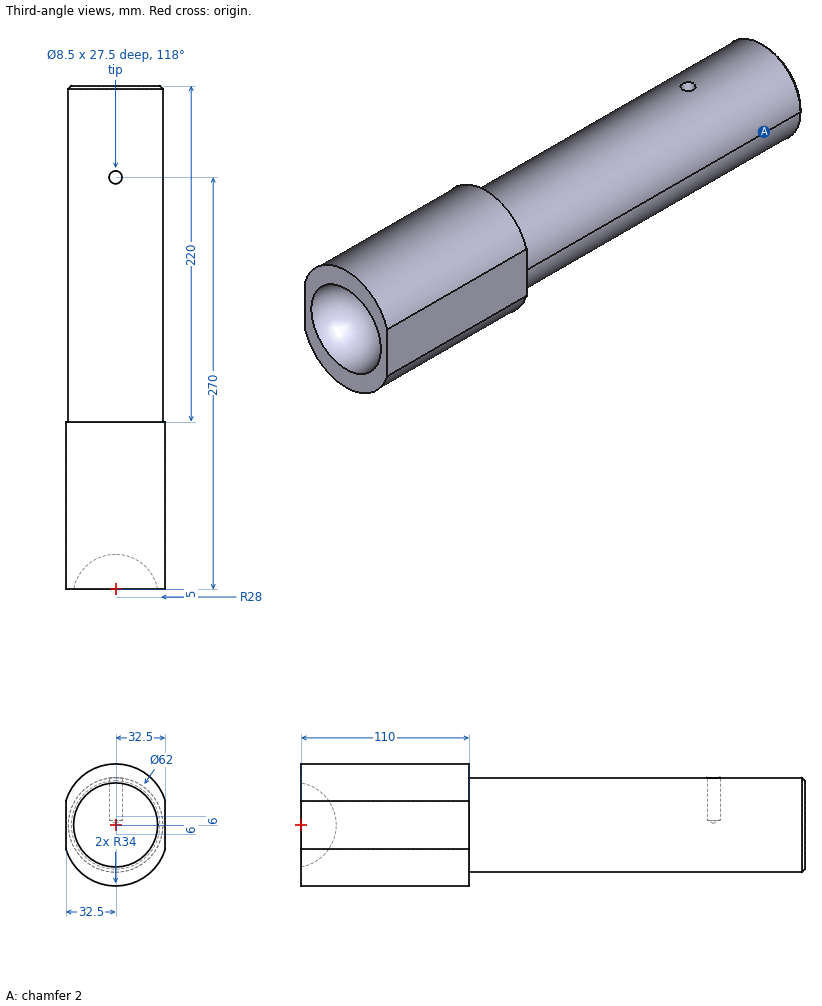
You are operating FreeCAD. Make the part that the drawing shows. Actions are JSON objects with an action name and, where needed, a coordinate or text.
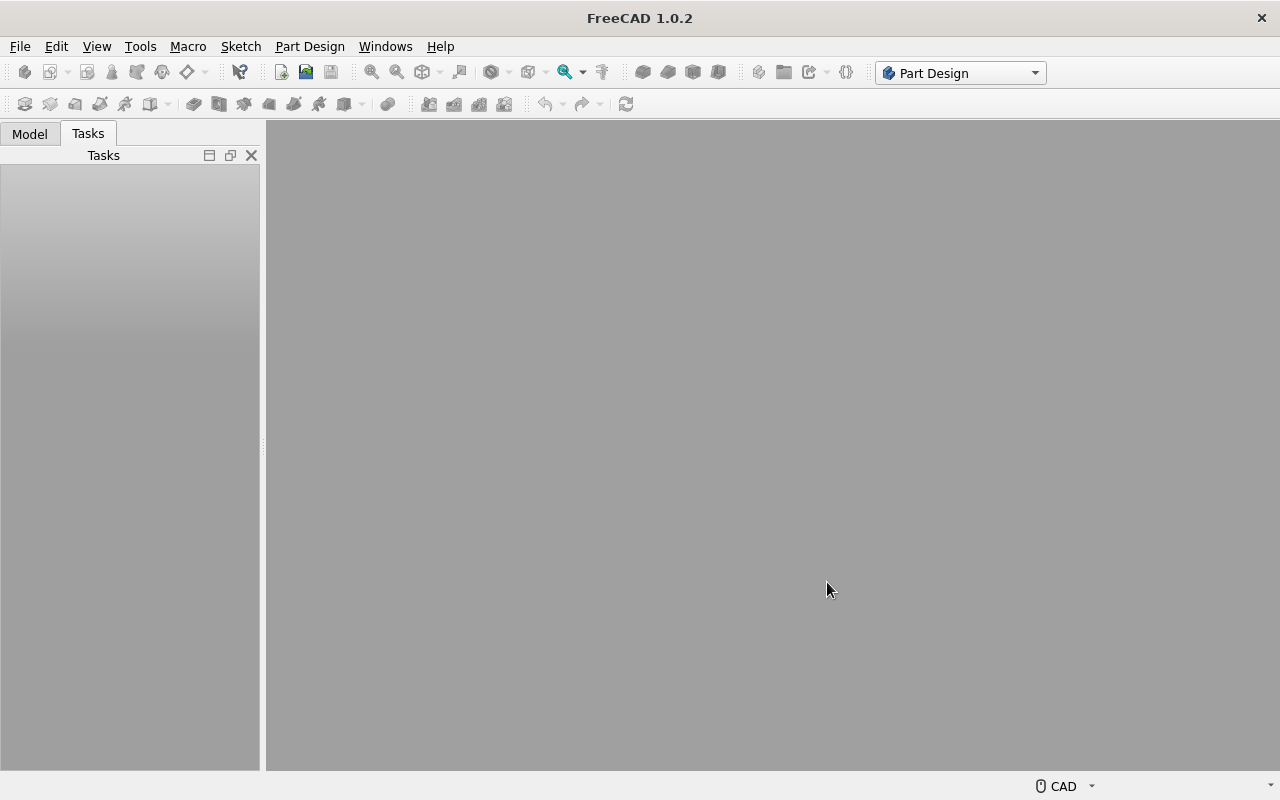
{"action": "left_click", "coordinate": [281, 72]}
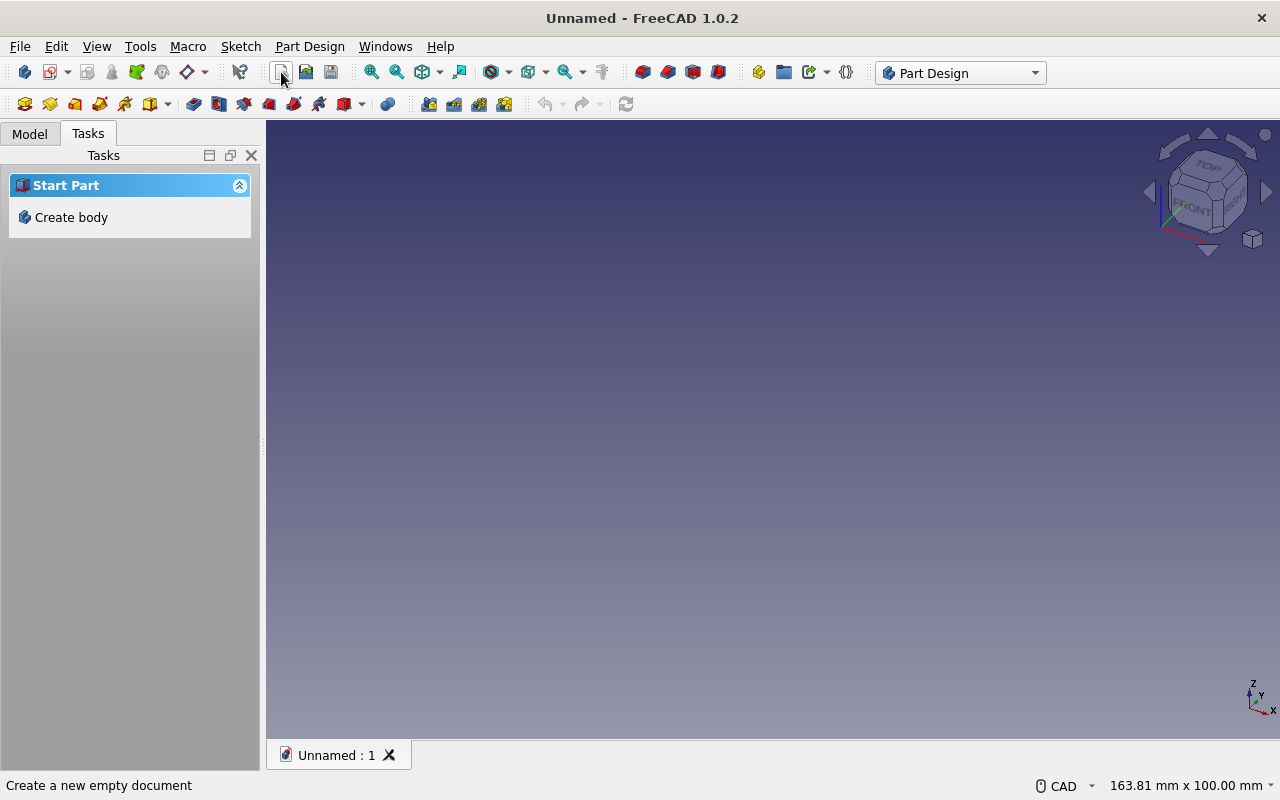
{"action": "left_click", "coordinate": [50, 72]}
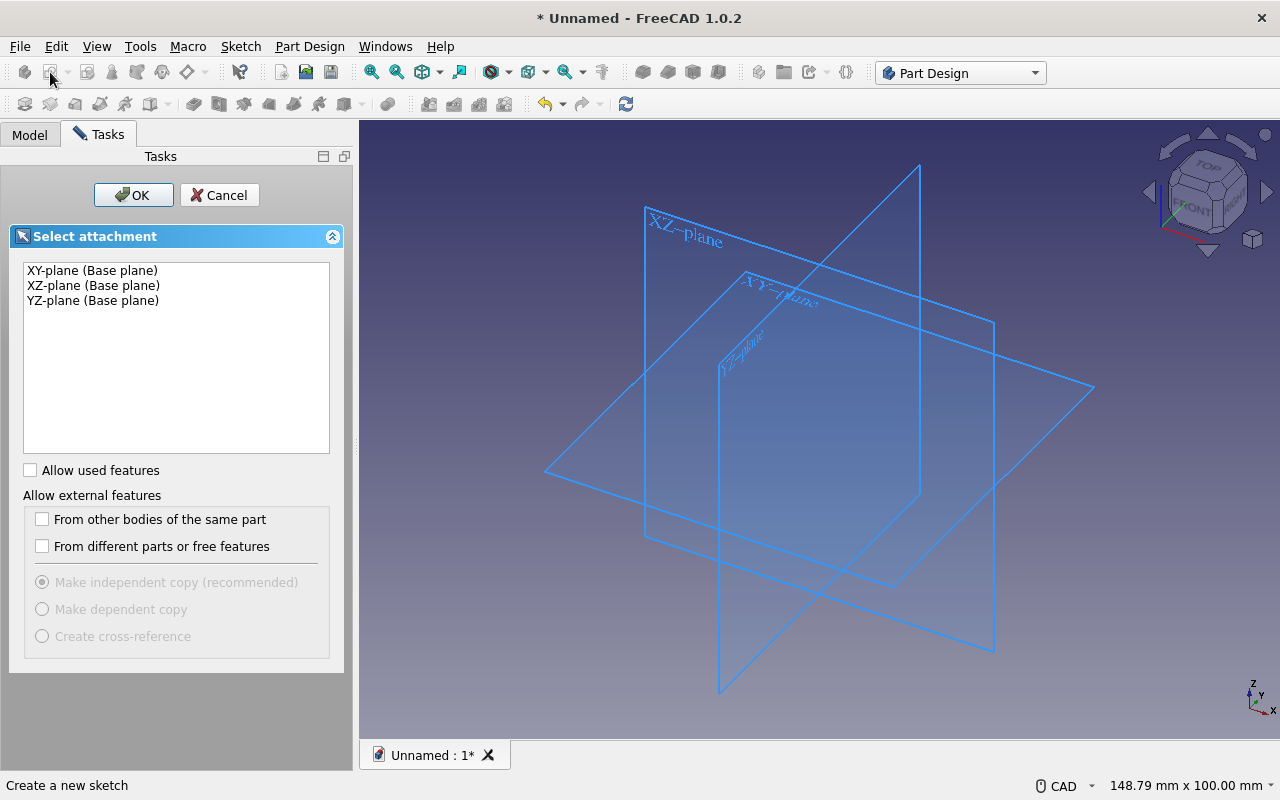
{"action": "left_click", "coordinate": [84, 286]}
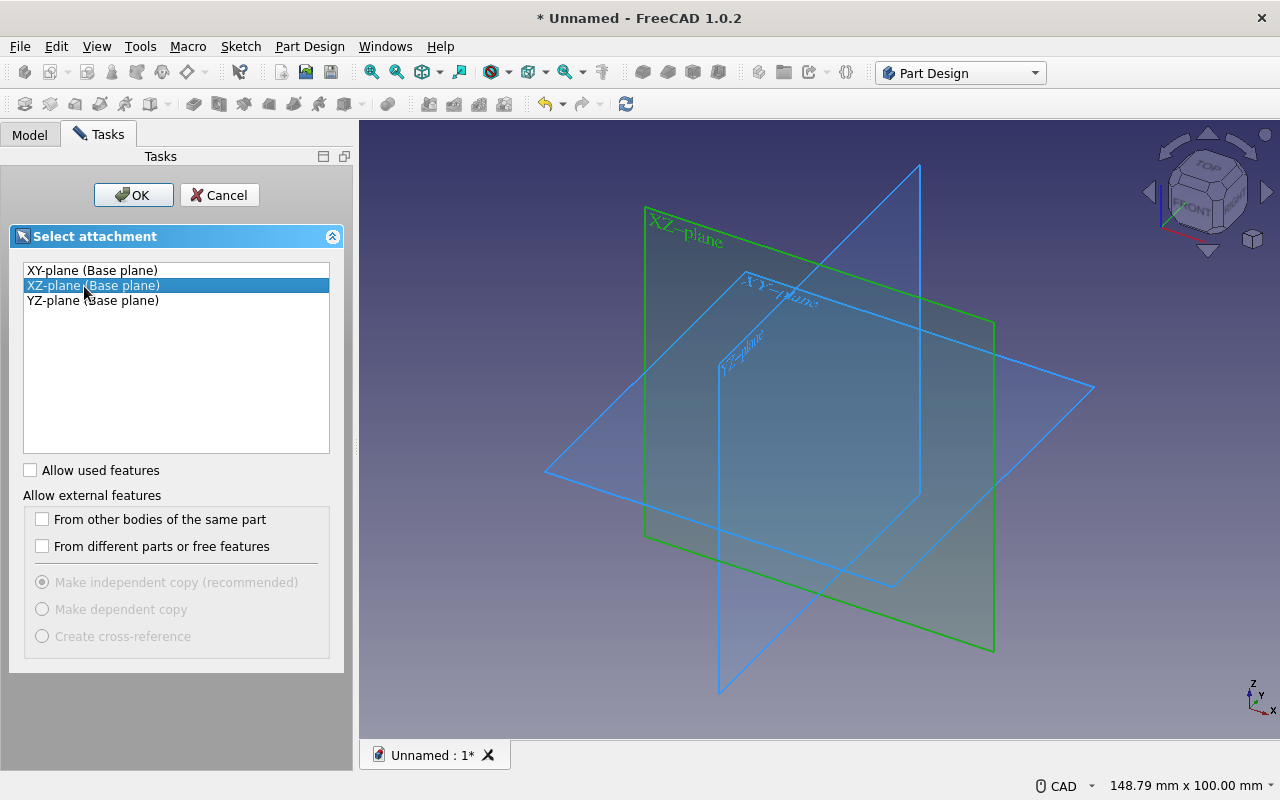
{"action": "left_click", "coordinate": [134, 195]}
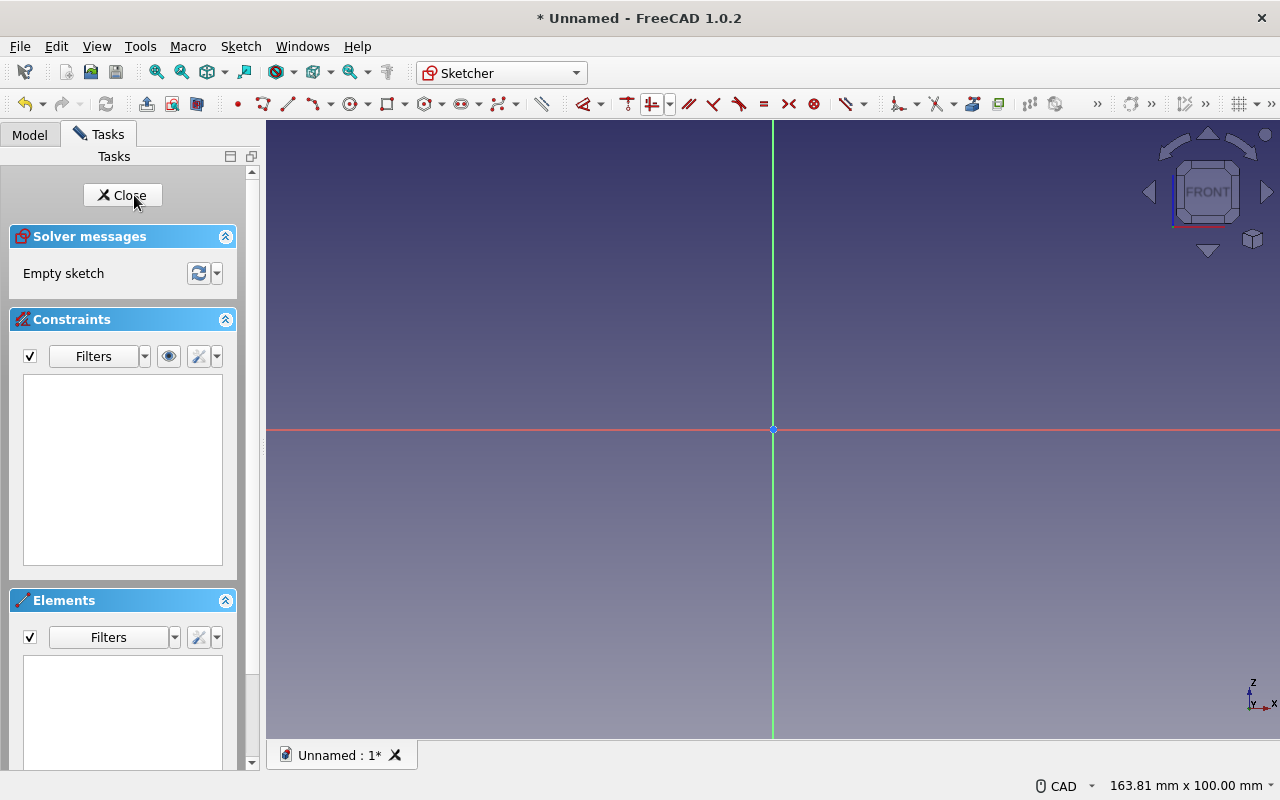
{"action": "left_click", "coordinate": [288, 104]}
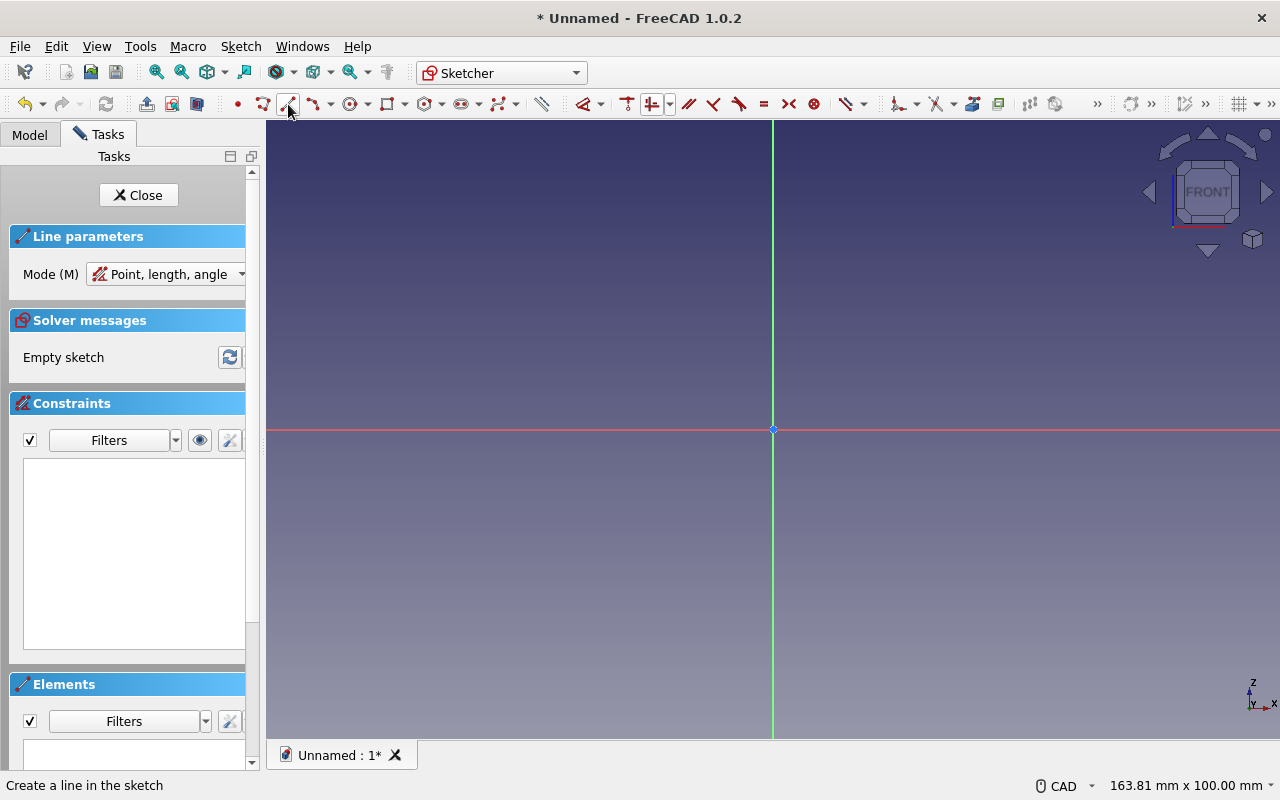
{"action": "left_click", "coordinate": [974, 331]}
{"action": "left_click", "coordinate": [974, 528]}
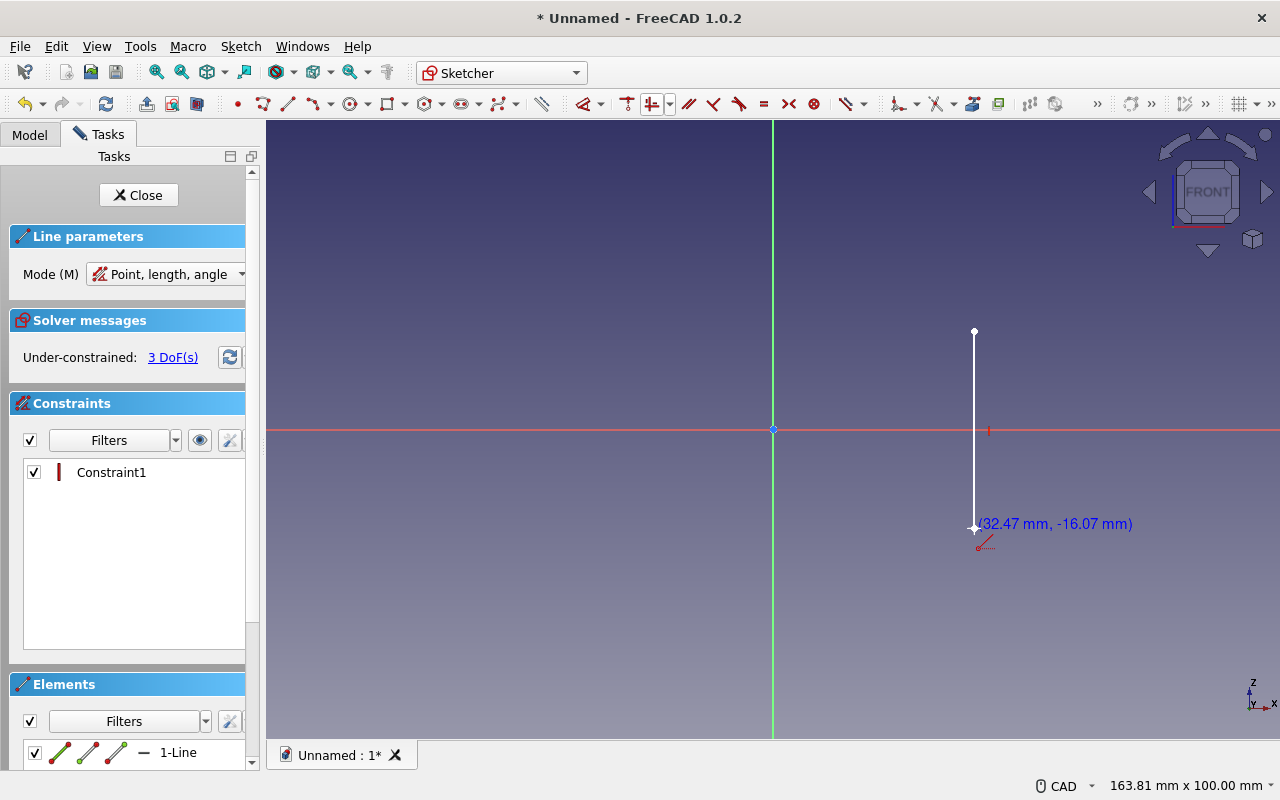
{"action": "left_click", "coordinate": [572, 528]}
{"action": "left_click", "coordinate": [572, 331]}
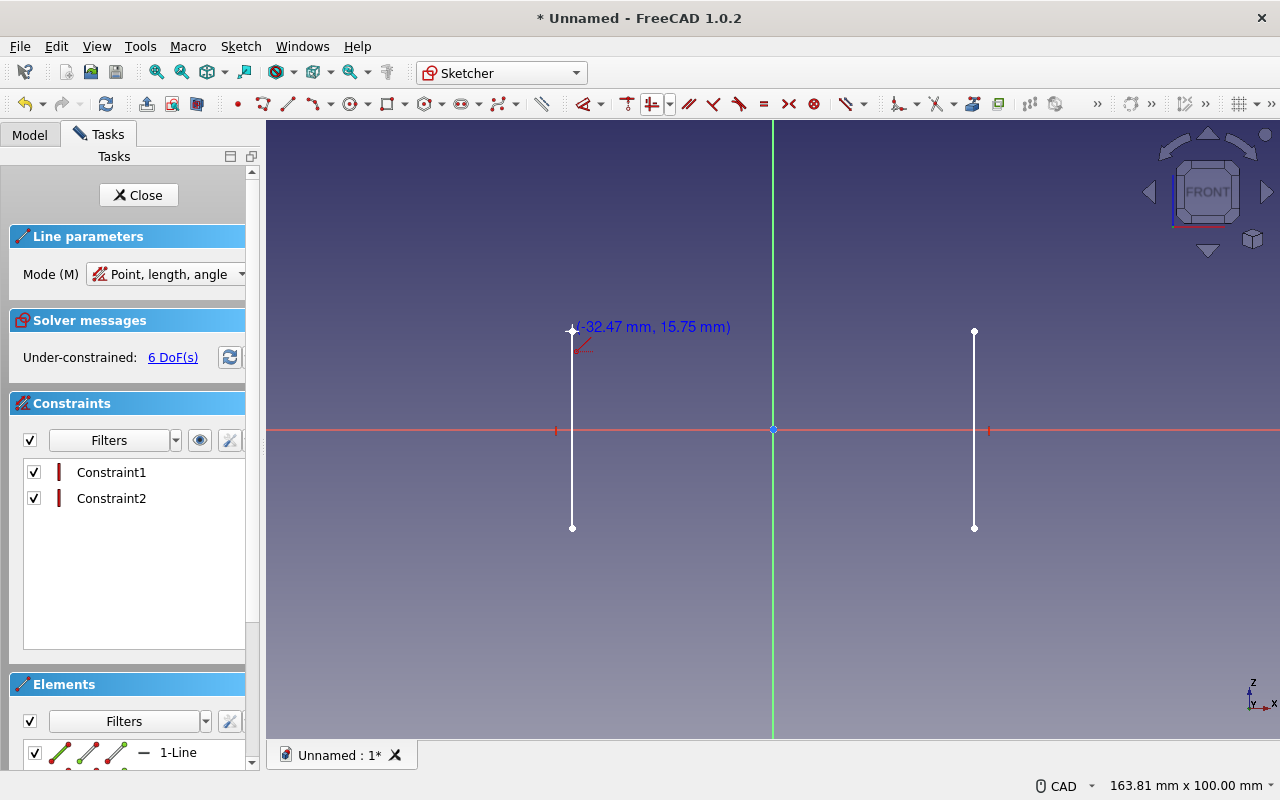
{"action": "left_click", "coordinate": [312, 104]}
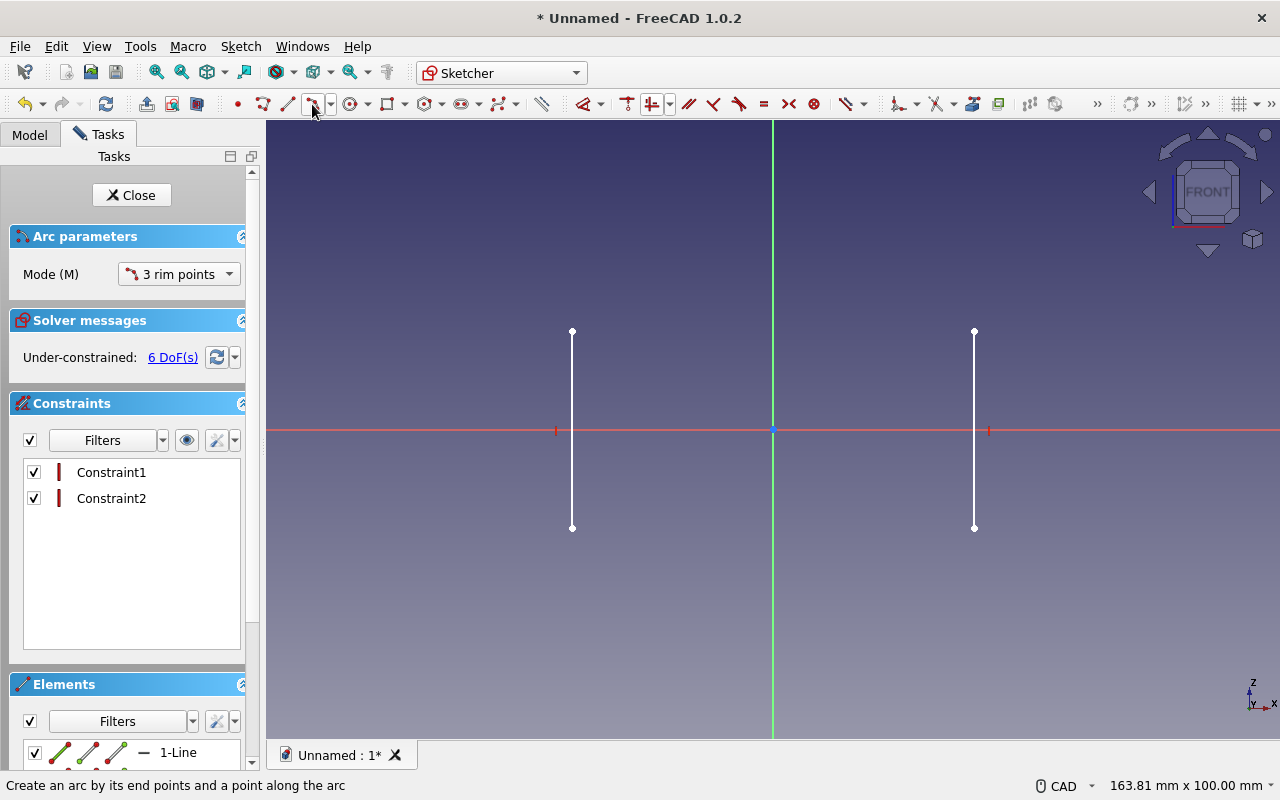
{"action": "left_click", "coordinate": [974, 529]}
{"action": "left_click", "coordinate": [572, 529]}
{"action": "left_click", "coordinate": [720, 670]}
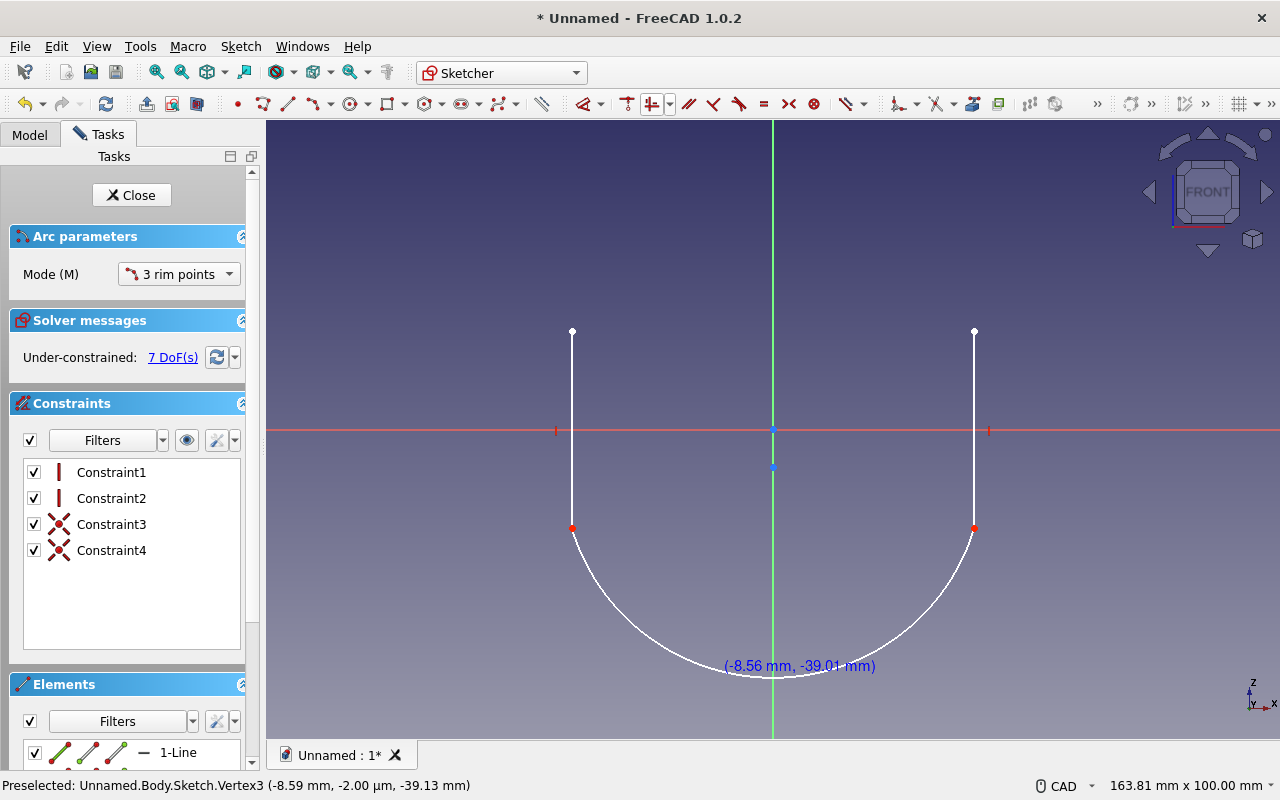
{"action": "left_click", "coordinate": [572, 332]}
{"action": "left_click", "coordinate": [974, 332]}
{"action": "left_click", "coordinate": [826, 189]}
{"action": "key", "text": "Escape"}